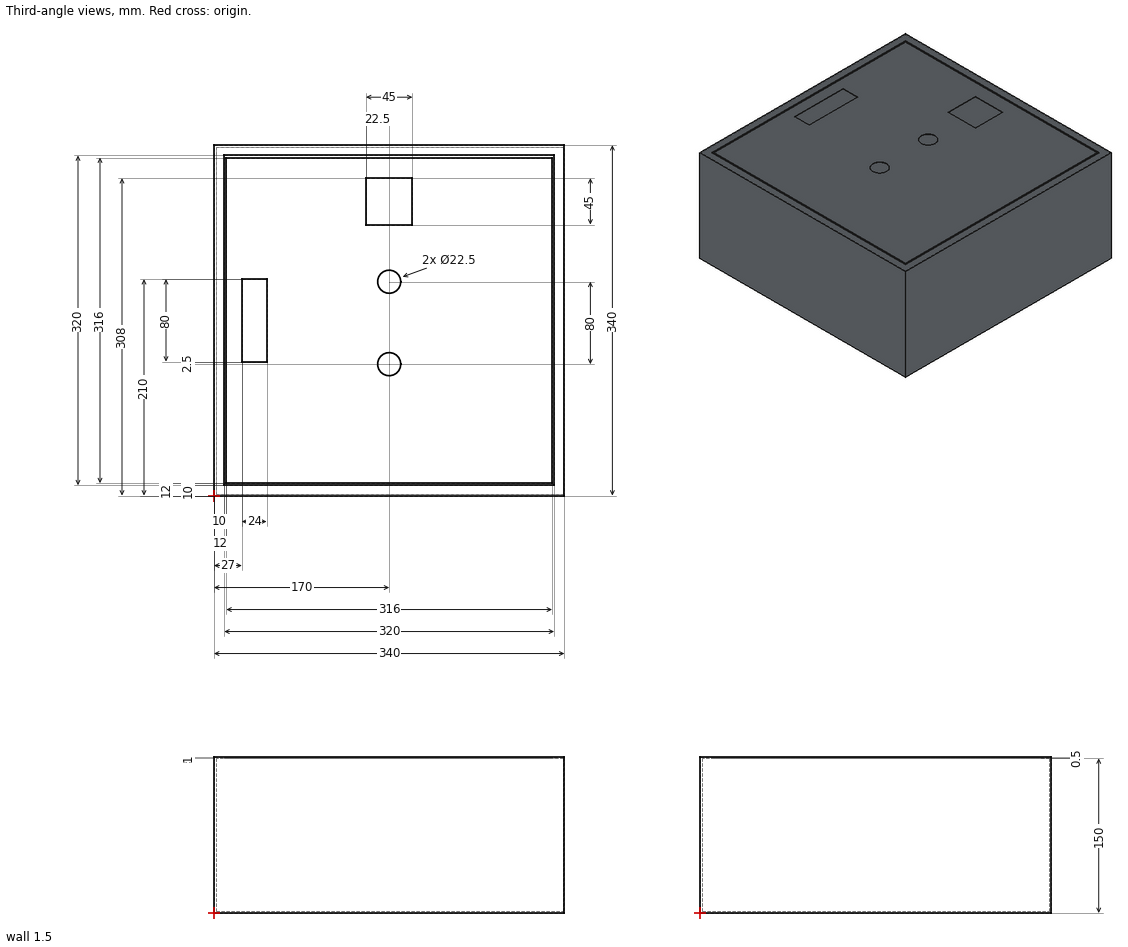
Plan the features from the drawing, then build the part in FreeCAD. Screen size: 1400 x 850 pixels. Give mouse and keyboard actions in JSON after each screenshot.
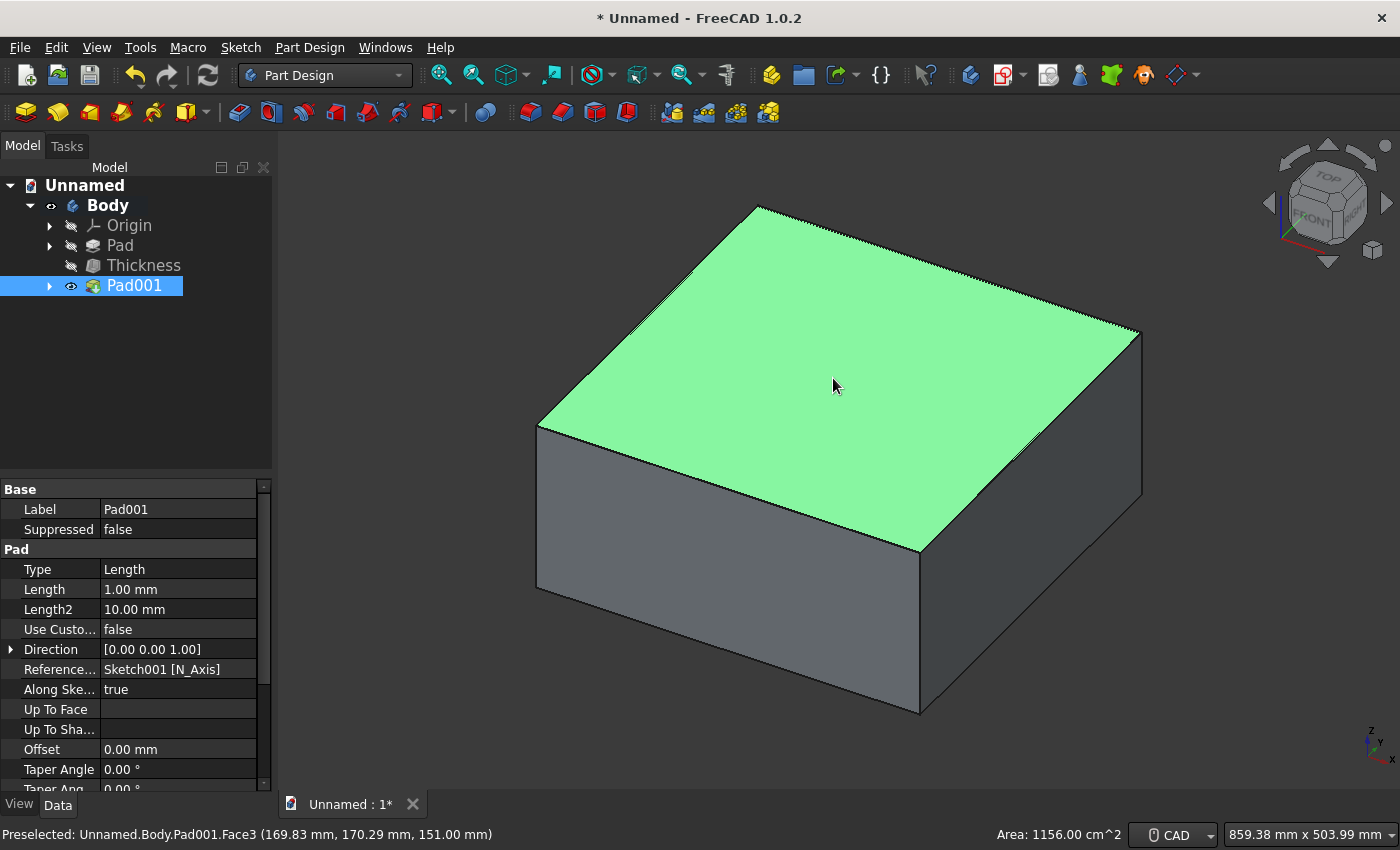
{"action": "left_click", "coordinate": [1004, 76]}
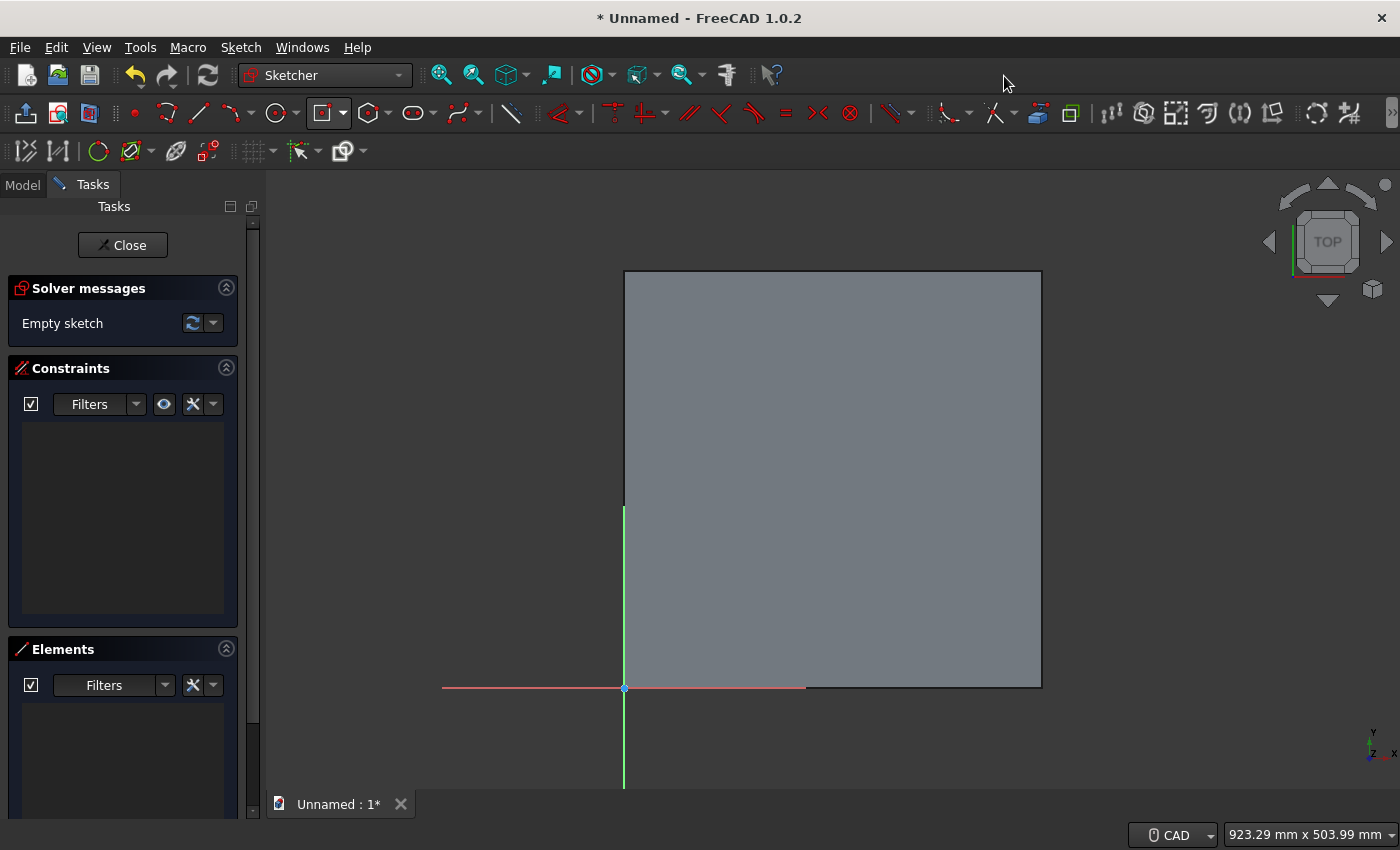
{"action": "key", "text": "g r"}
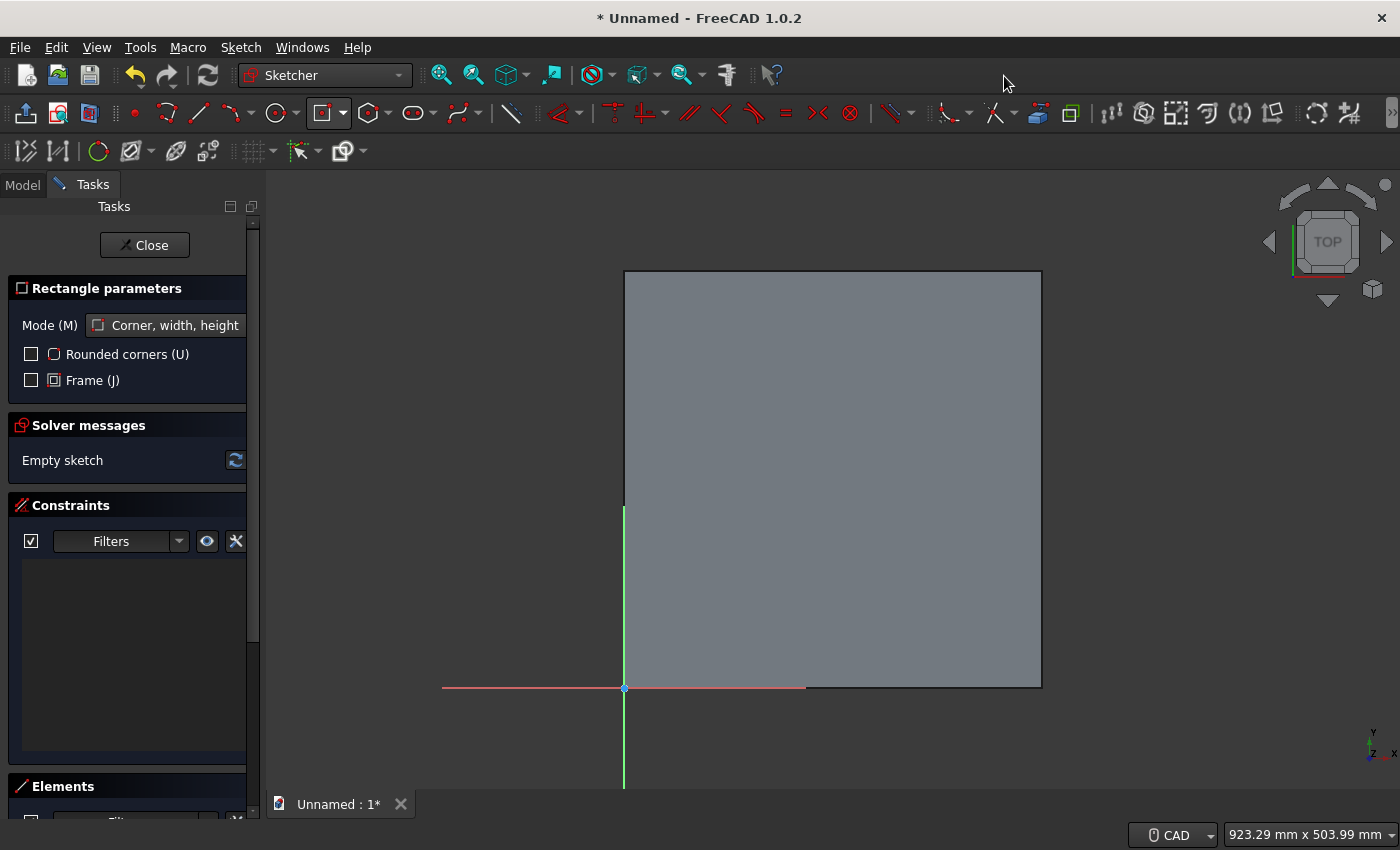
{"action": "scroll", "coordinate": [636, 283], "scroll_direction": "up", "scroll_amount": 2}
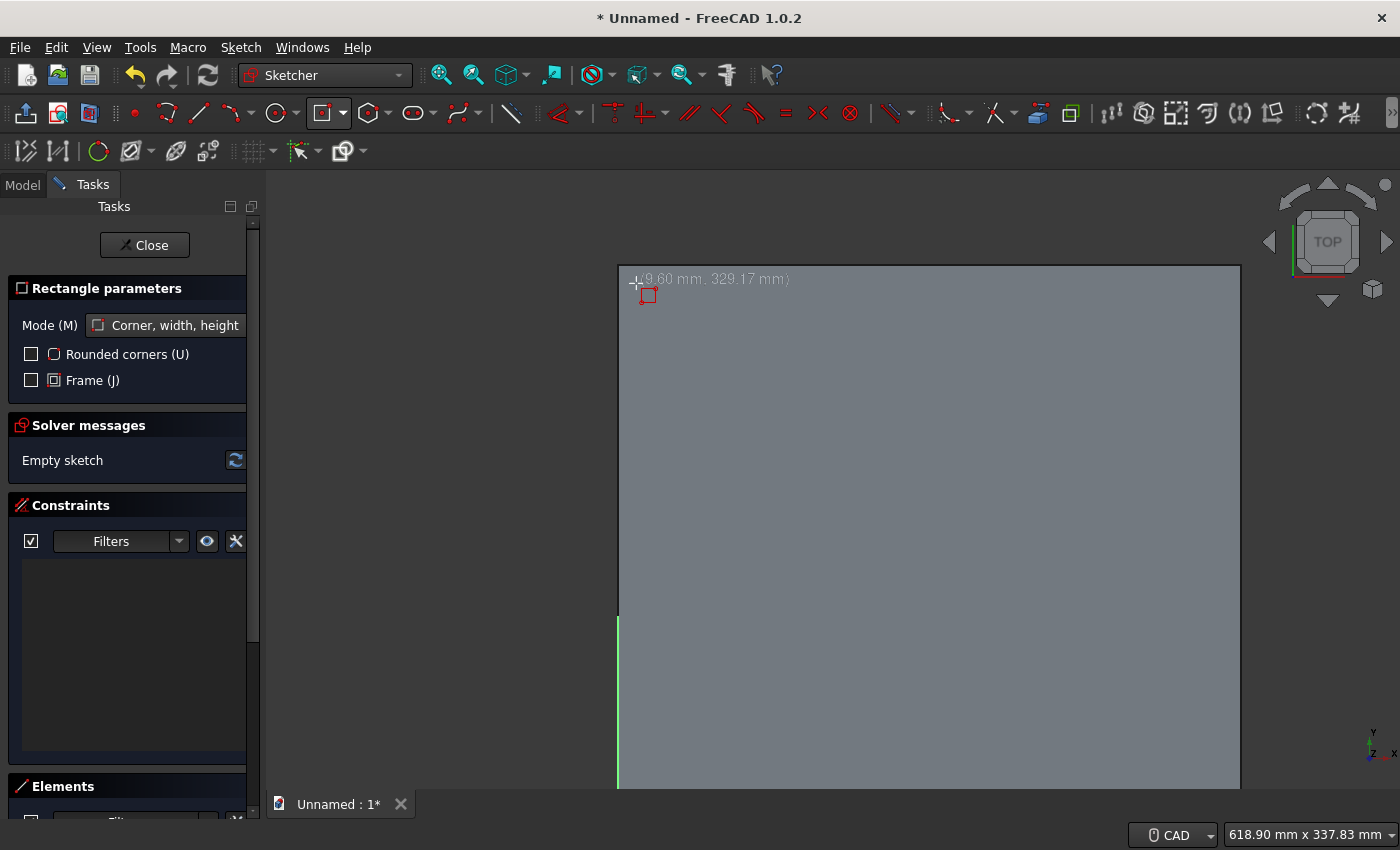
{"action": "left_click", "coordinate": [637, 283]}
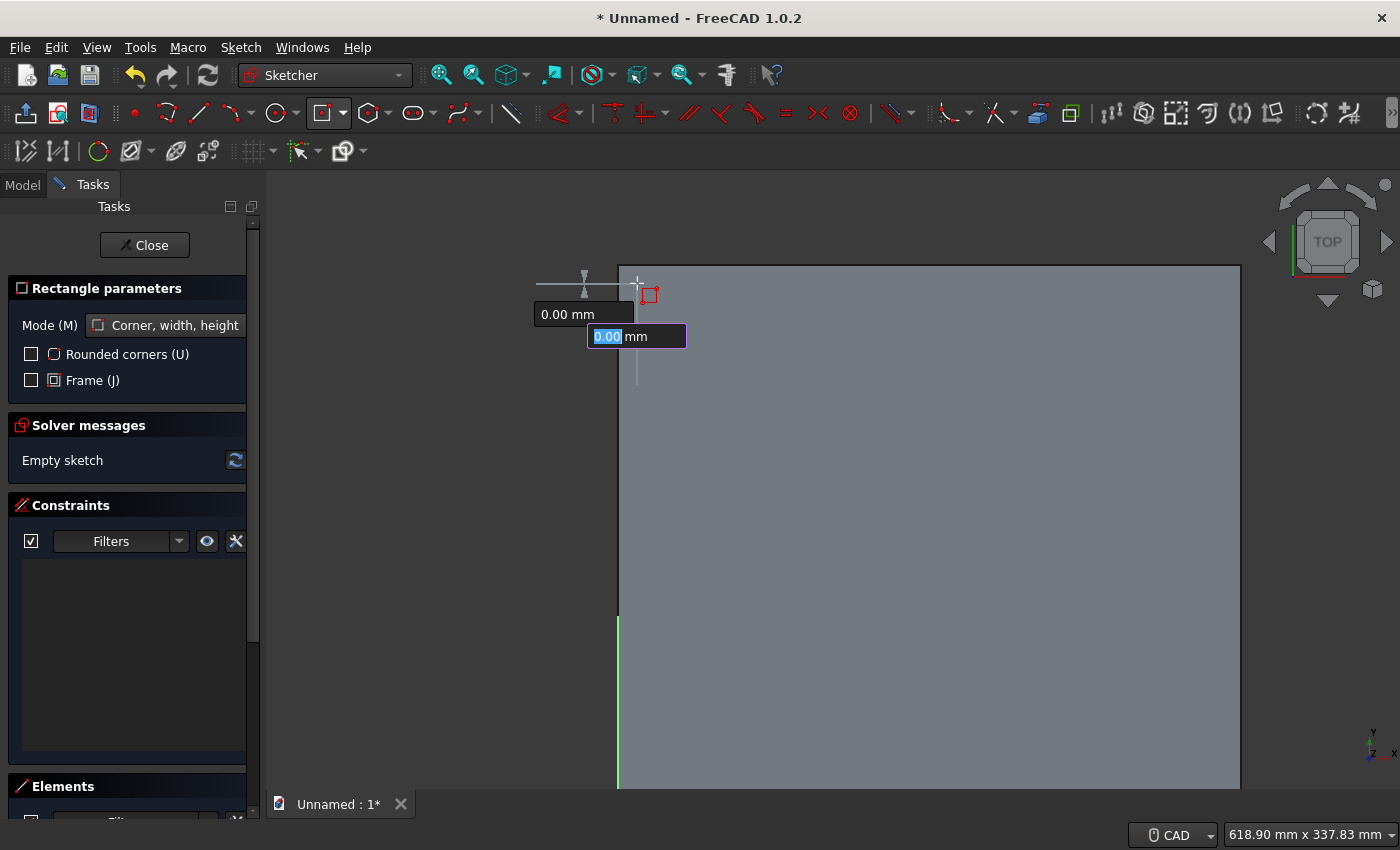
{"action": "scroll", "coordinate": [447, 265], "scroll_direction": "down", "scroll_amount": 2}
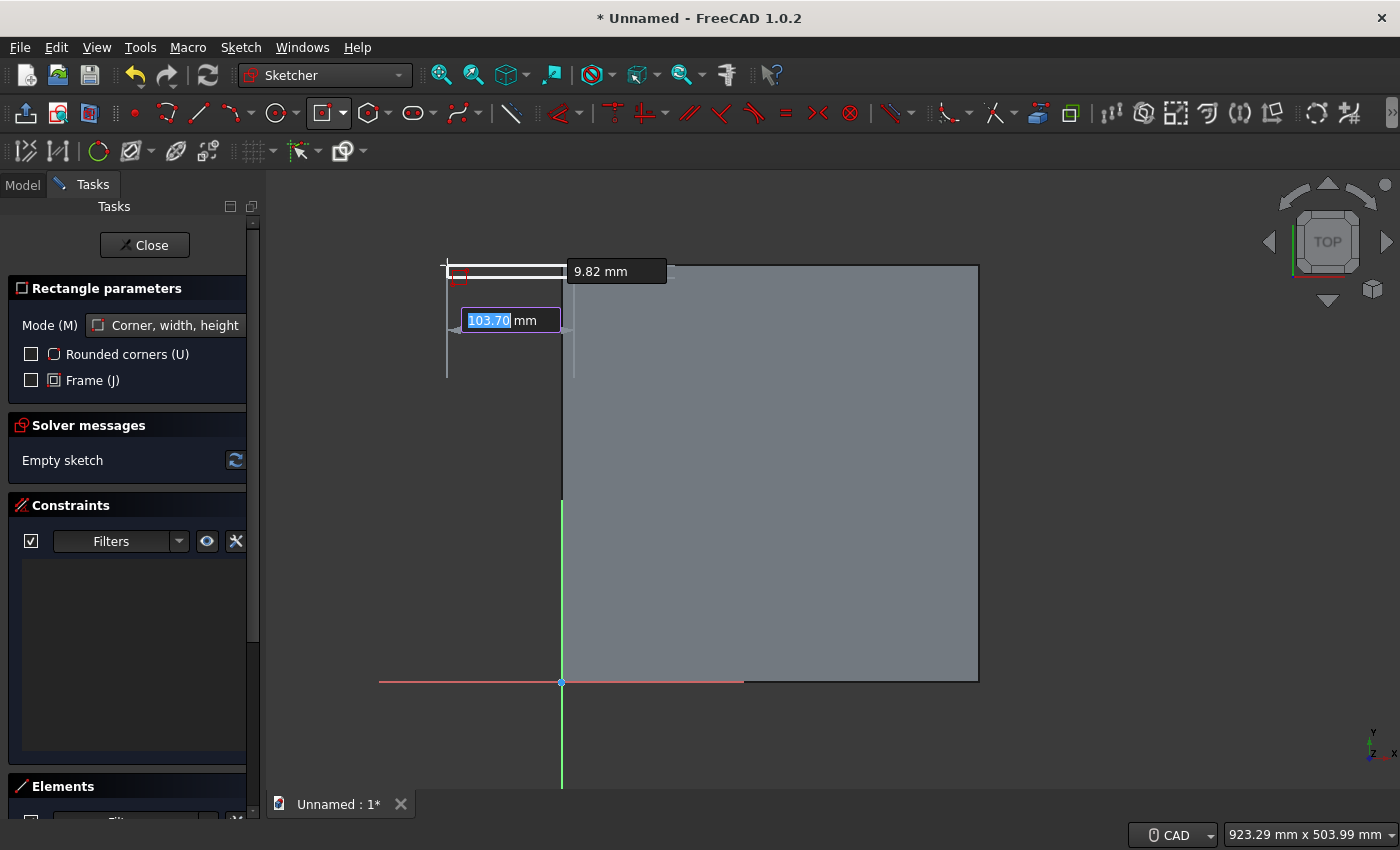
{"action": "scroll", "coordinate": [967, 670], "scroll_direction": "up", "scroll_amount": 2}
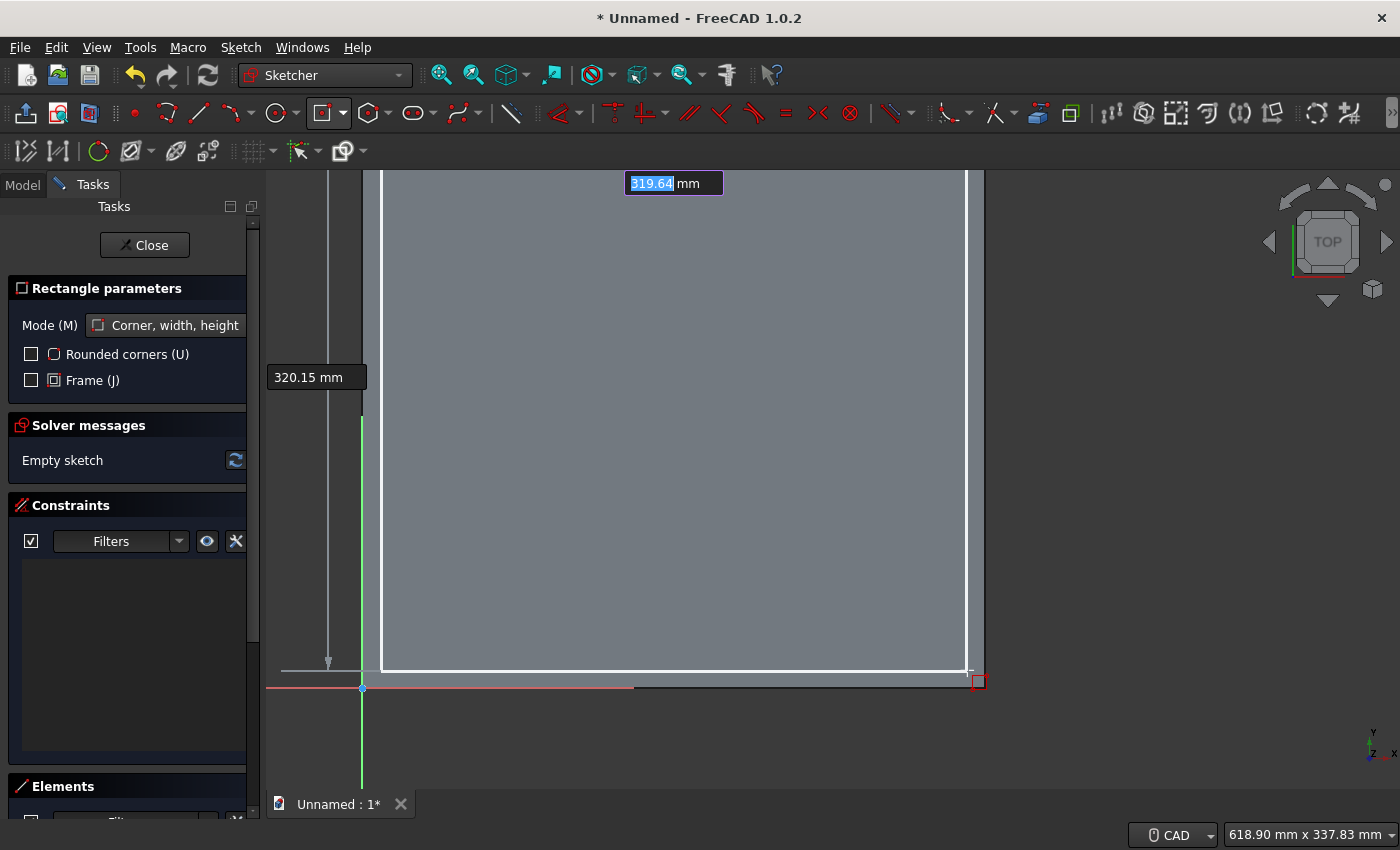
{"action": "left_click", "coordinate": [967, 670]}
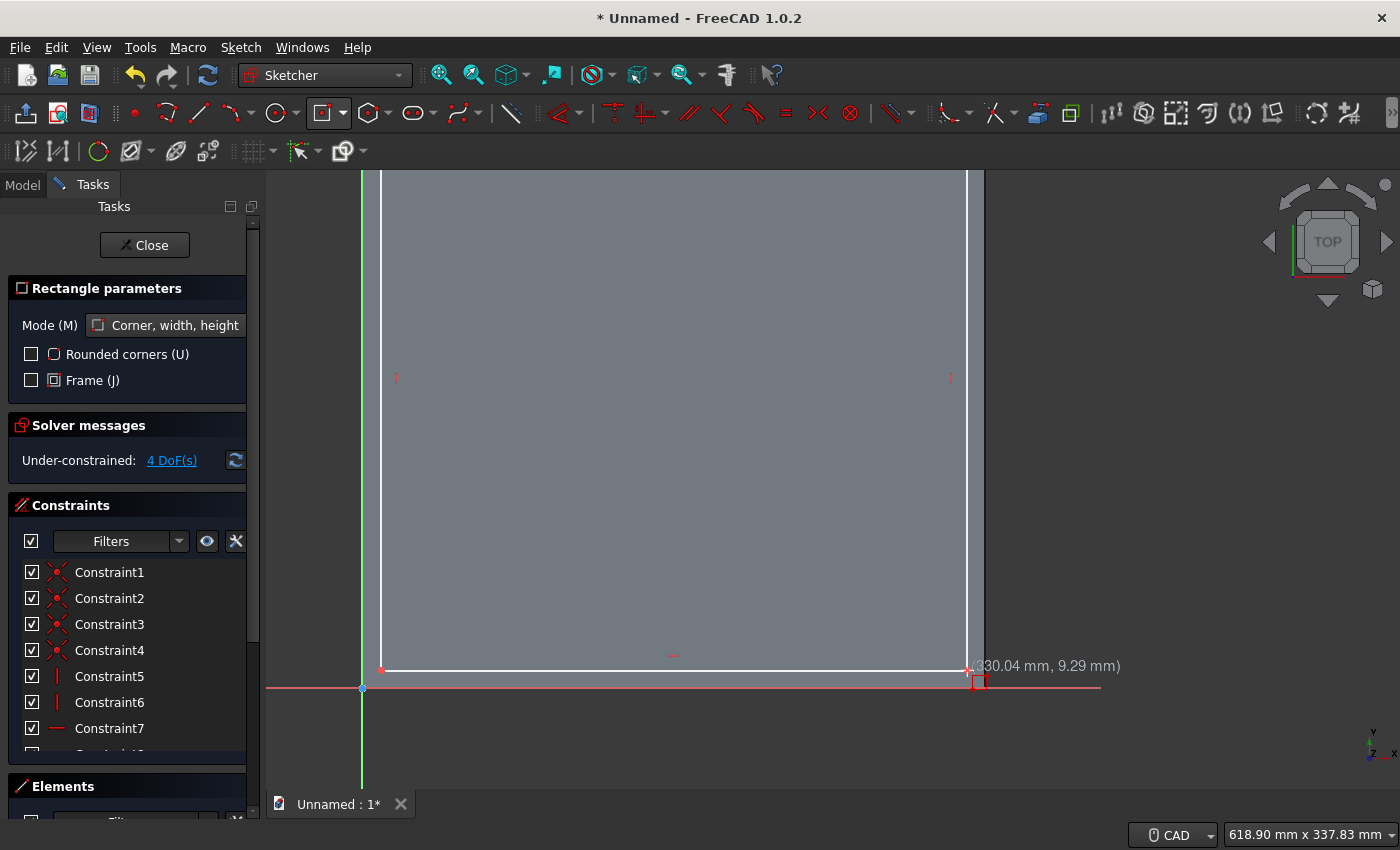
{"action": "left_click", "coordinate": [412, 303]}
{"action": "mouse_move", "coordinate": [456, 450]}